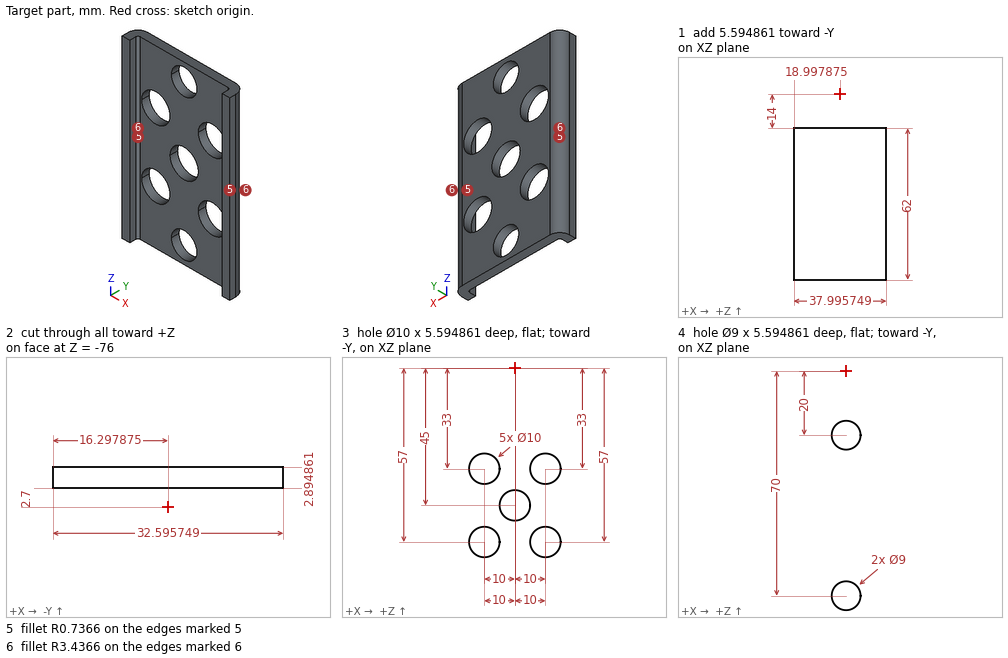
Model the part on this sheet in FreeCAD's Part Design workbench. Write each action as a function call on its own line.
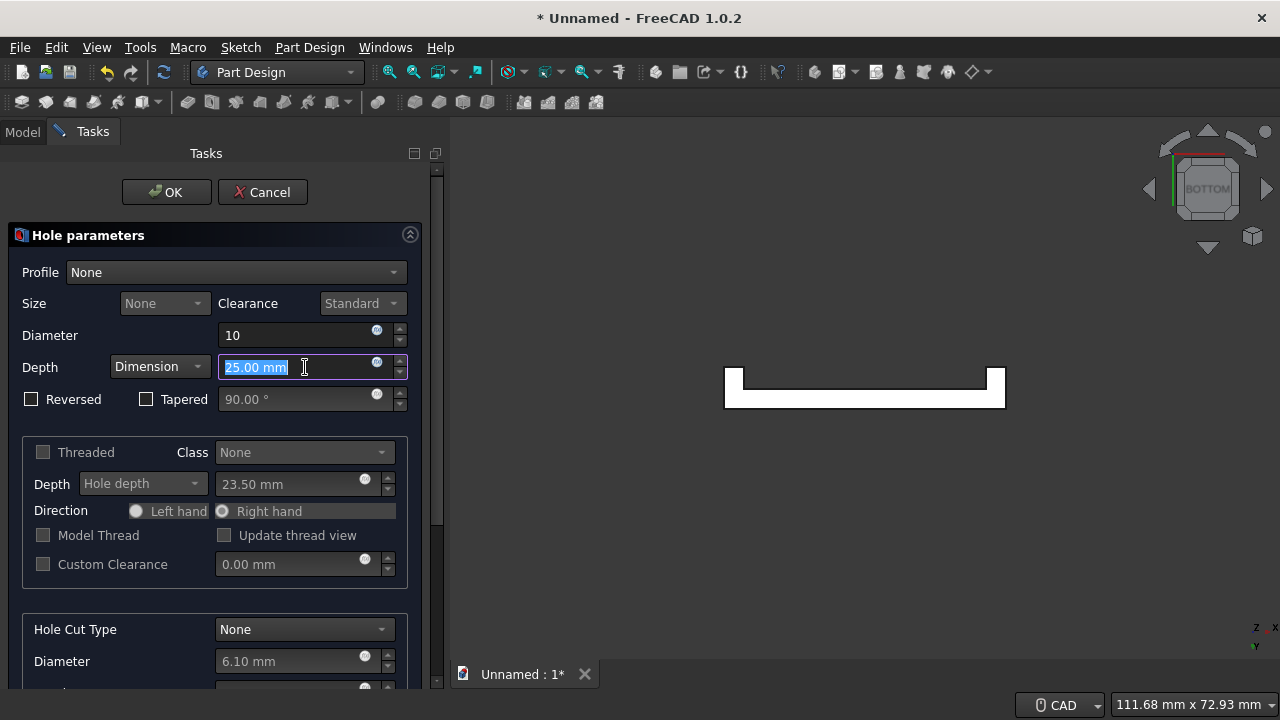
text(5.594861)
key(Tab)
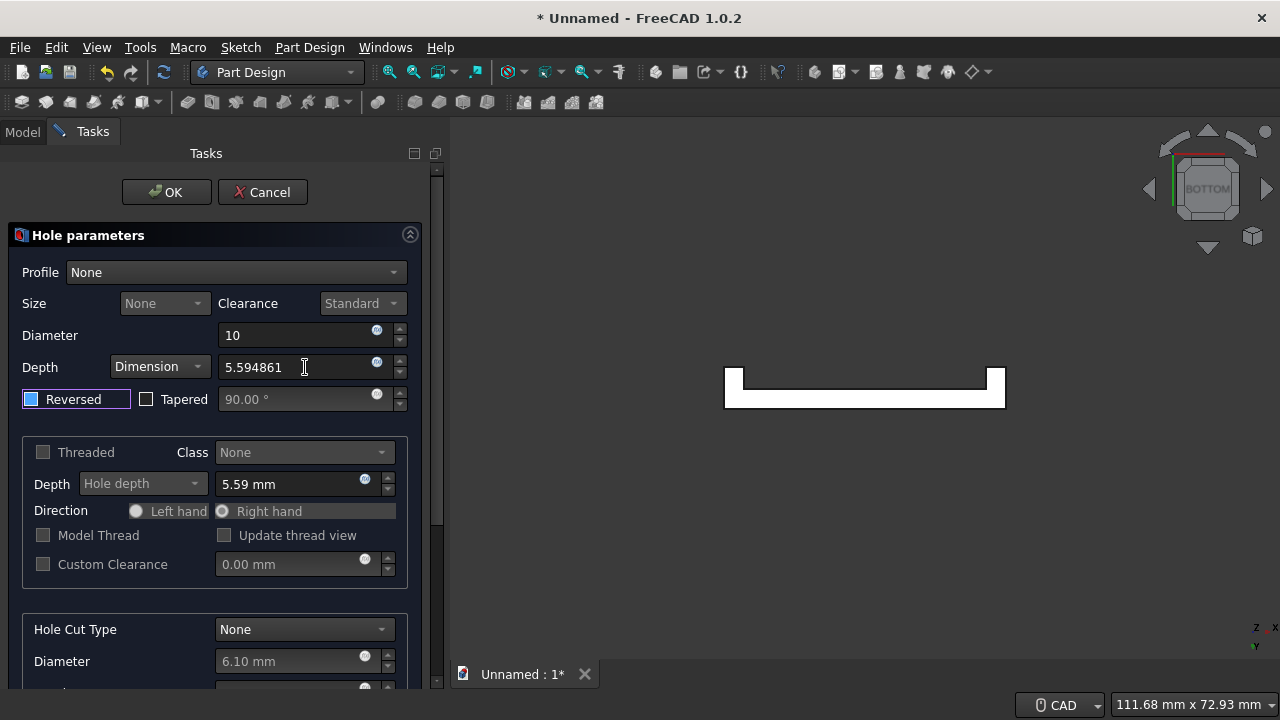
click(30, 399)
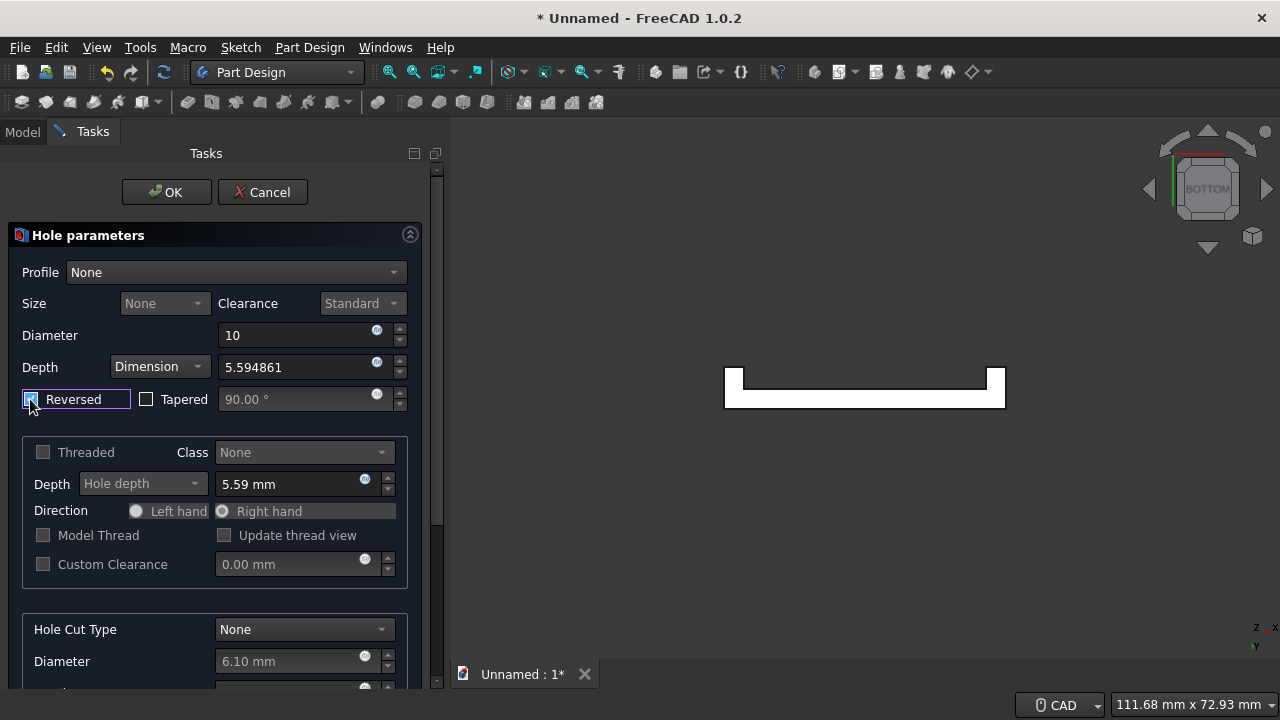
scroll(437, 426, down, 4)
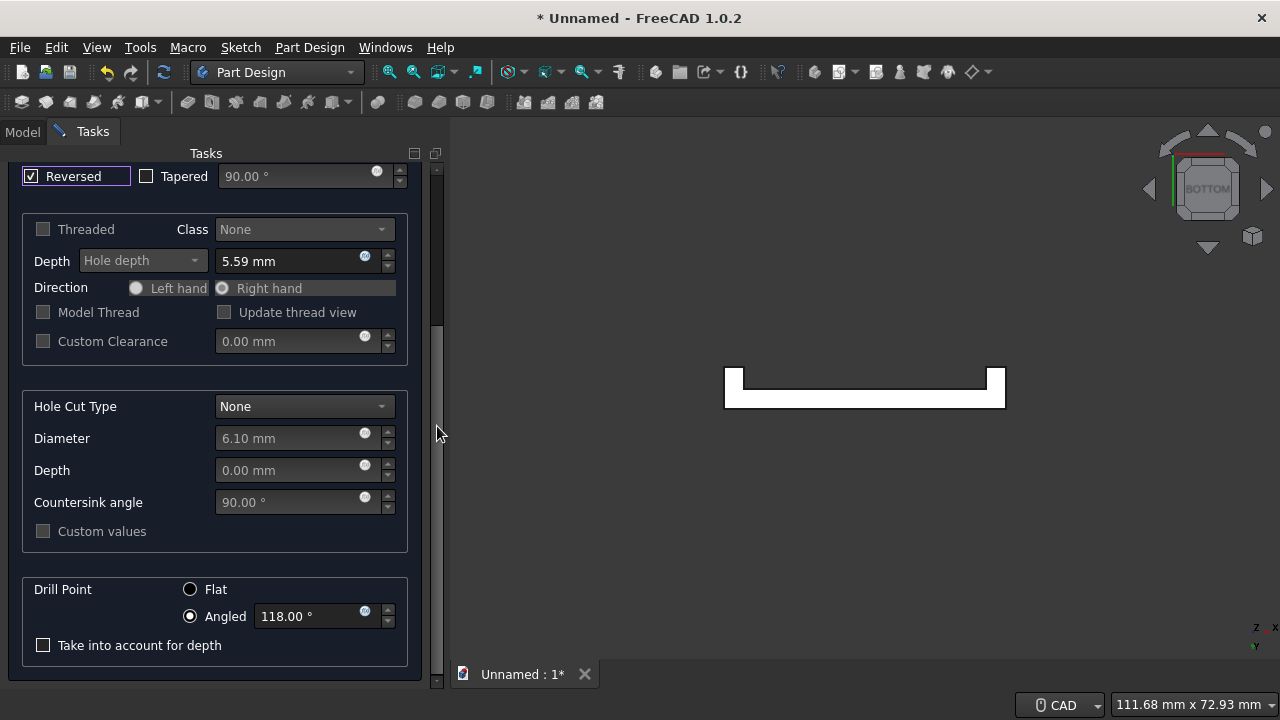
click(191, 589)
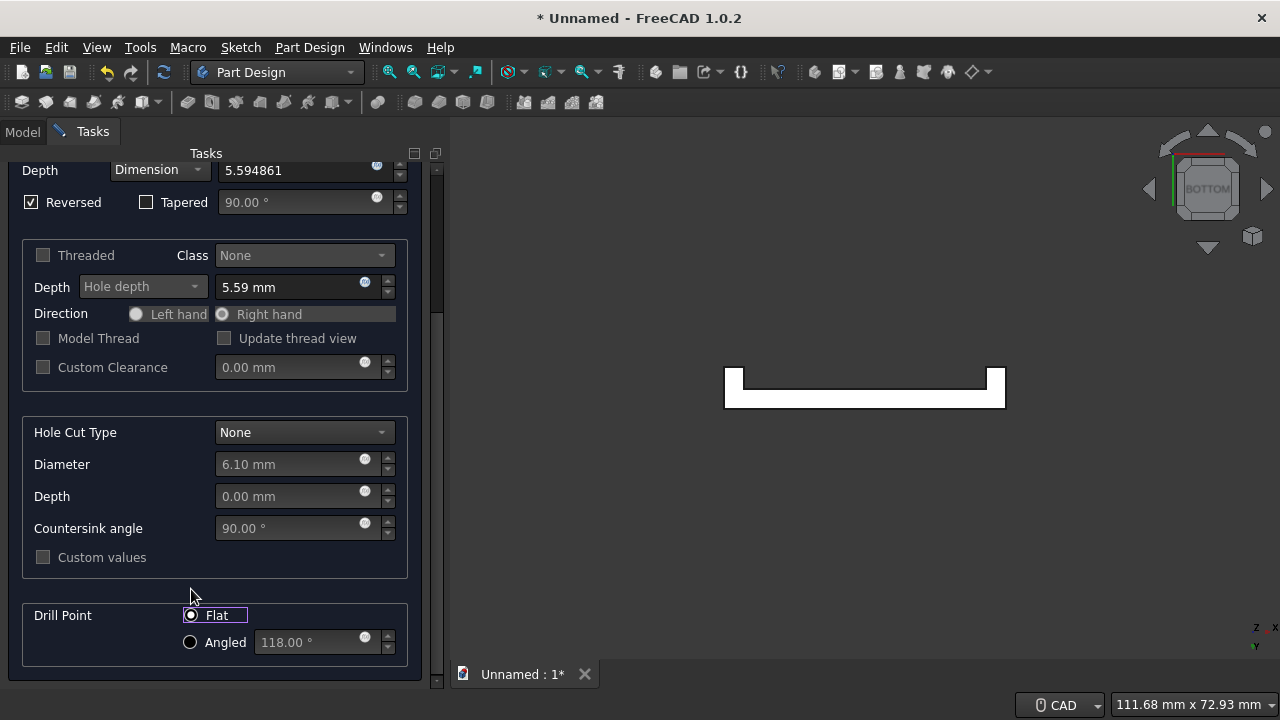
scroll(437, 426, up, 5)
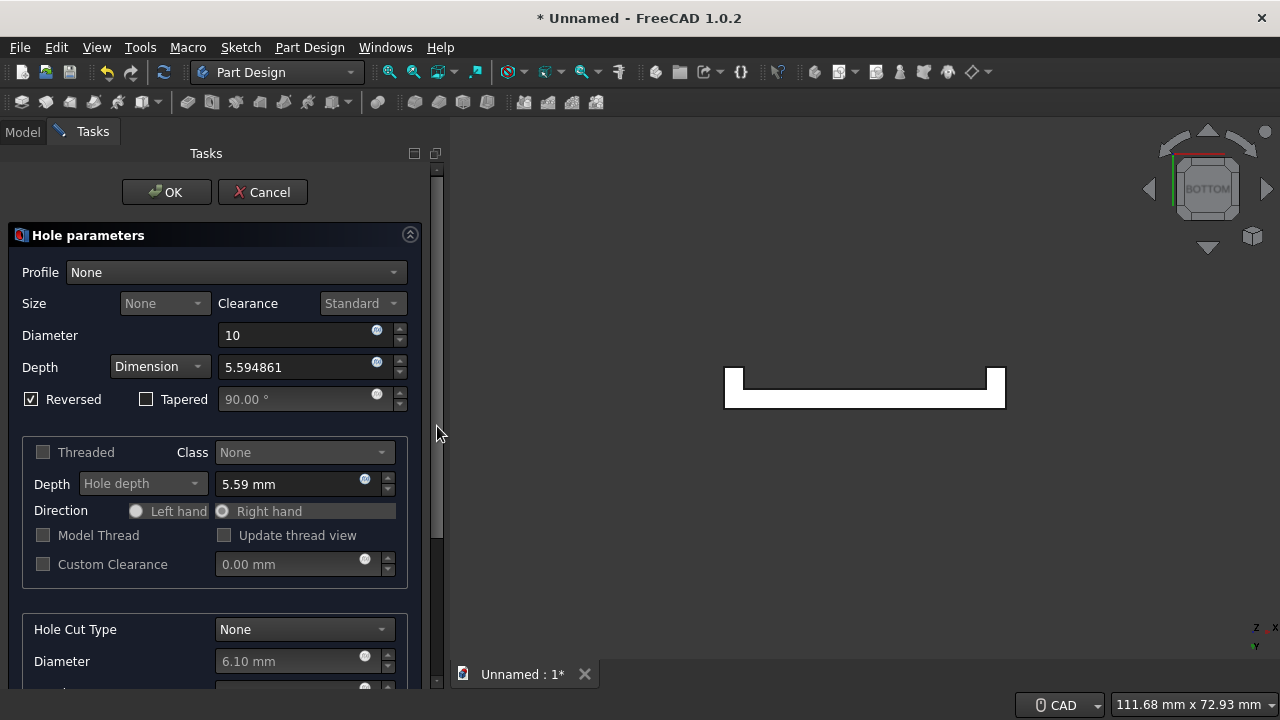
click(167, 192)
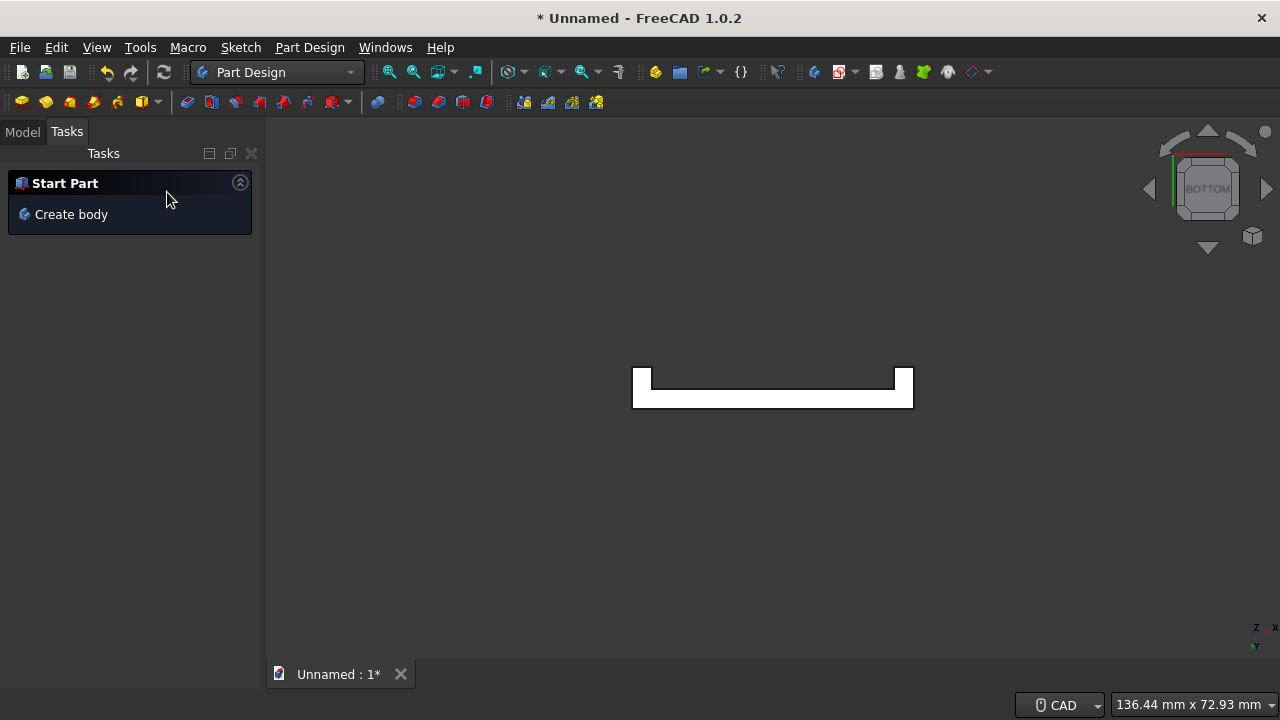
key(v)
key(f)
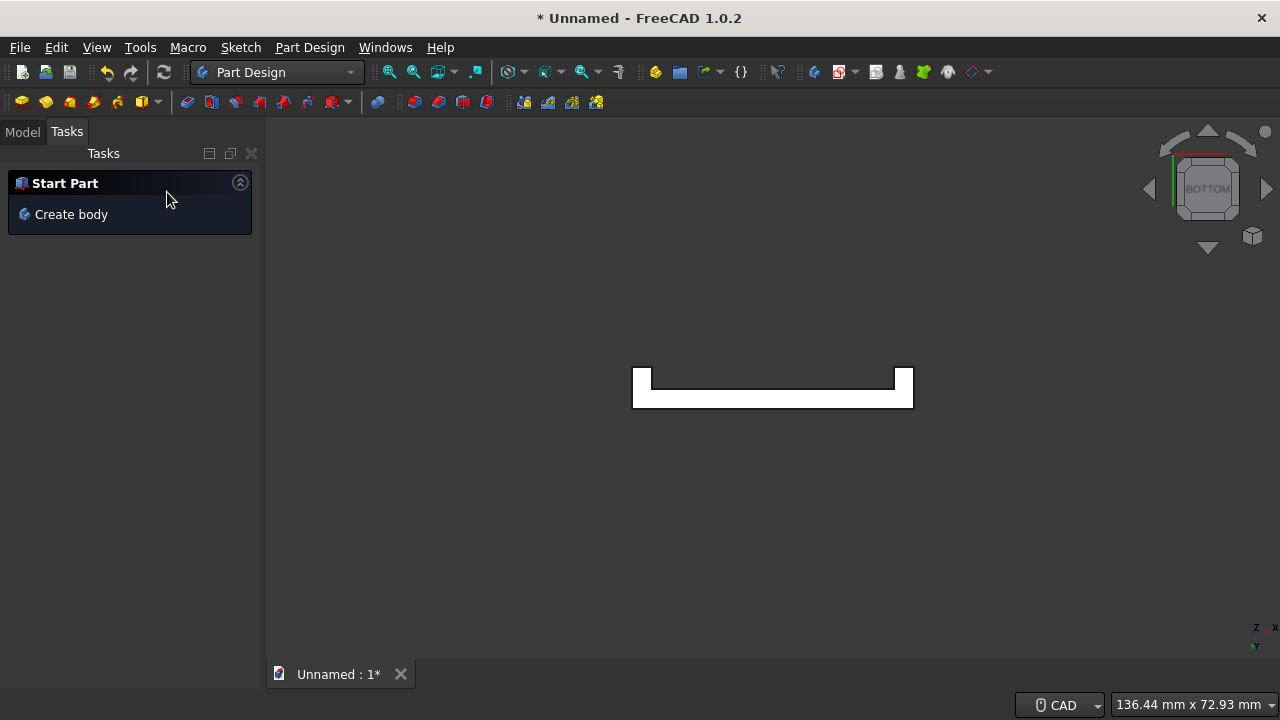
click(840, 72)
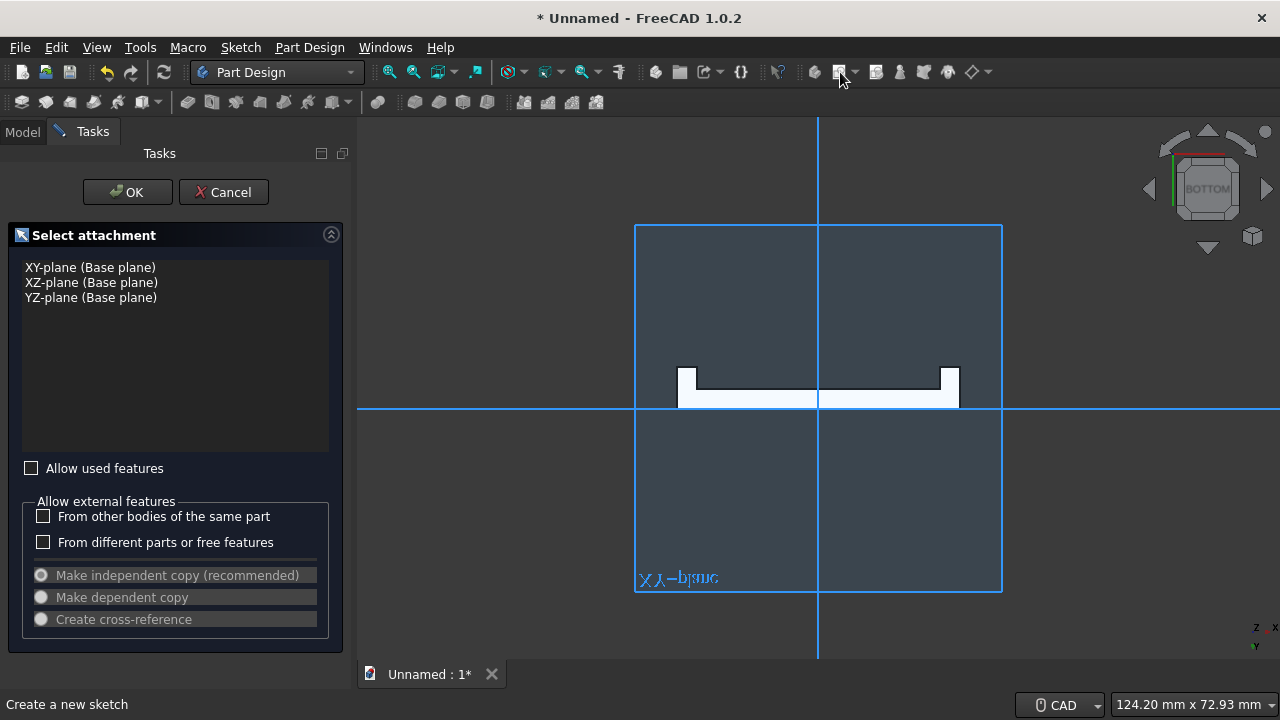
click(82, 282)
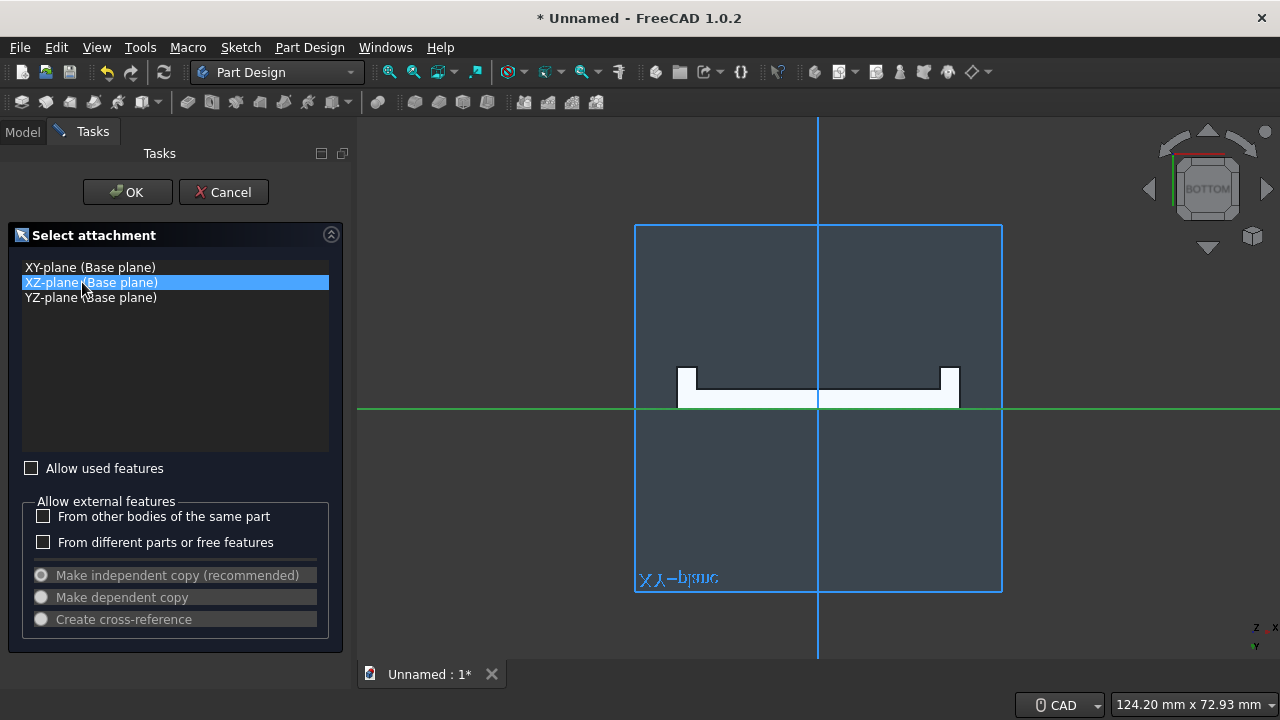
click(128, 192)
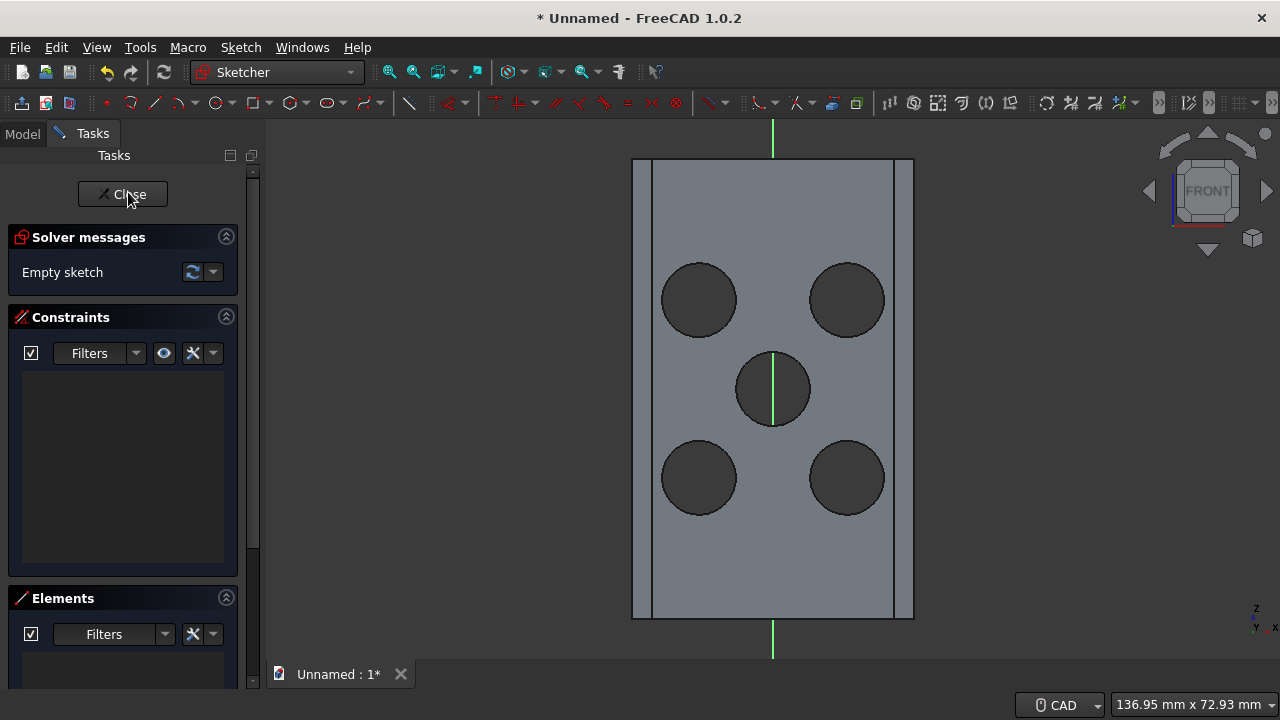
click(70, 104)